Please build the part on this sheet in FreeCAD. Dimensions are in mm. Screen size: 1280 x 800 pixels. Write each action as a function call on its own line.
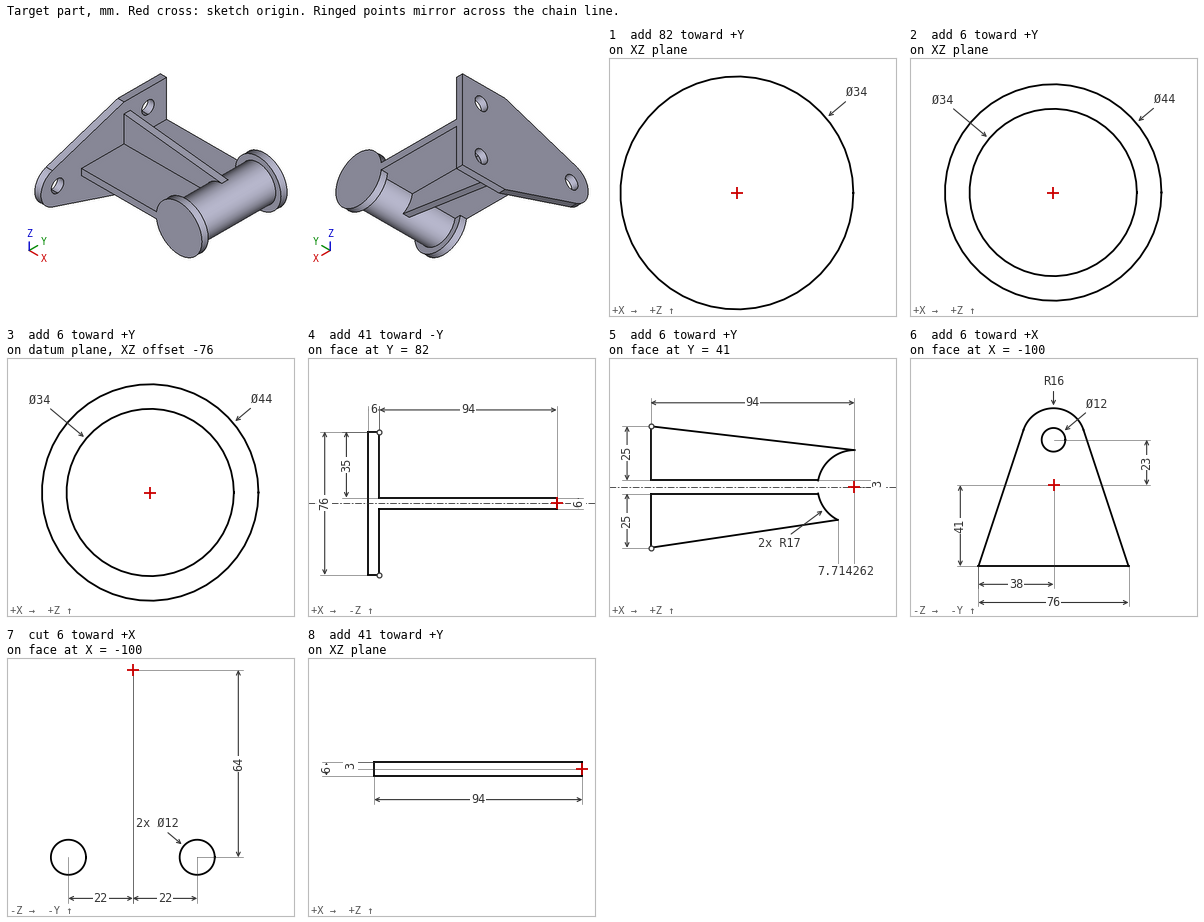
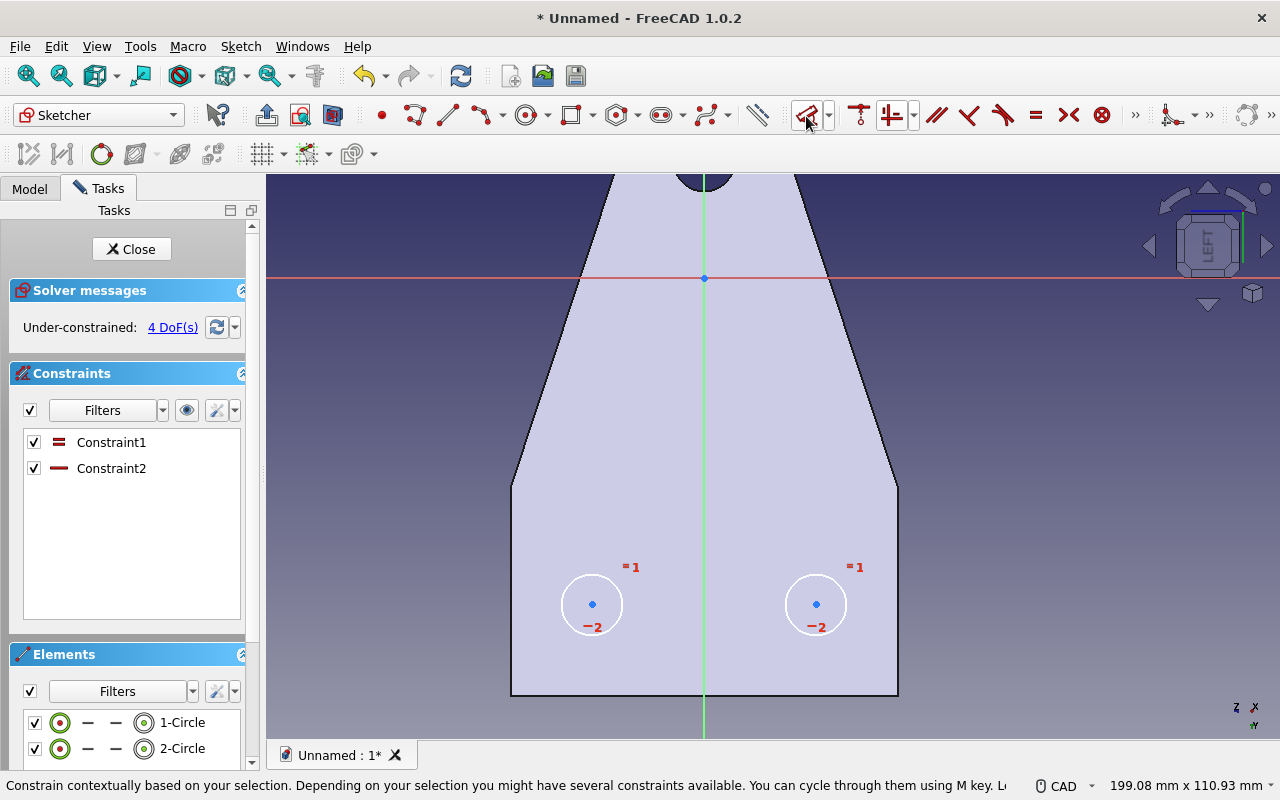
click(837, 583)
click(859, 560)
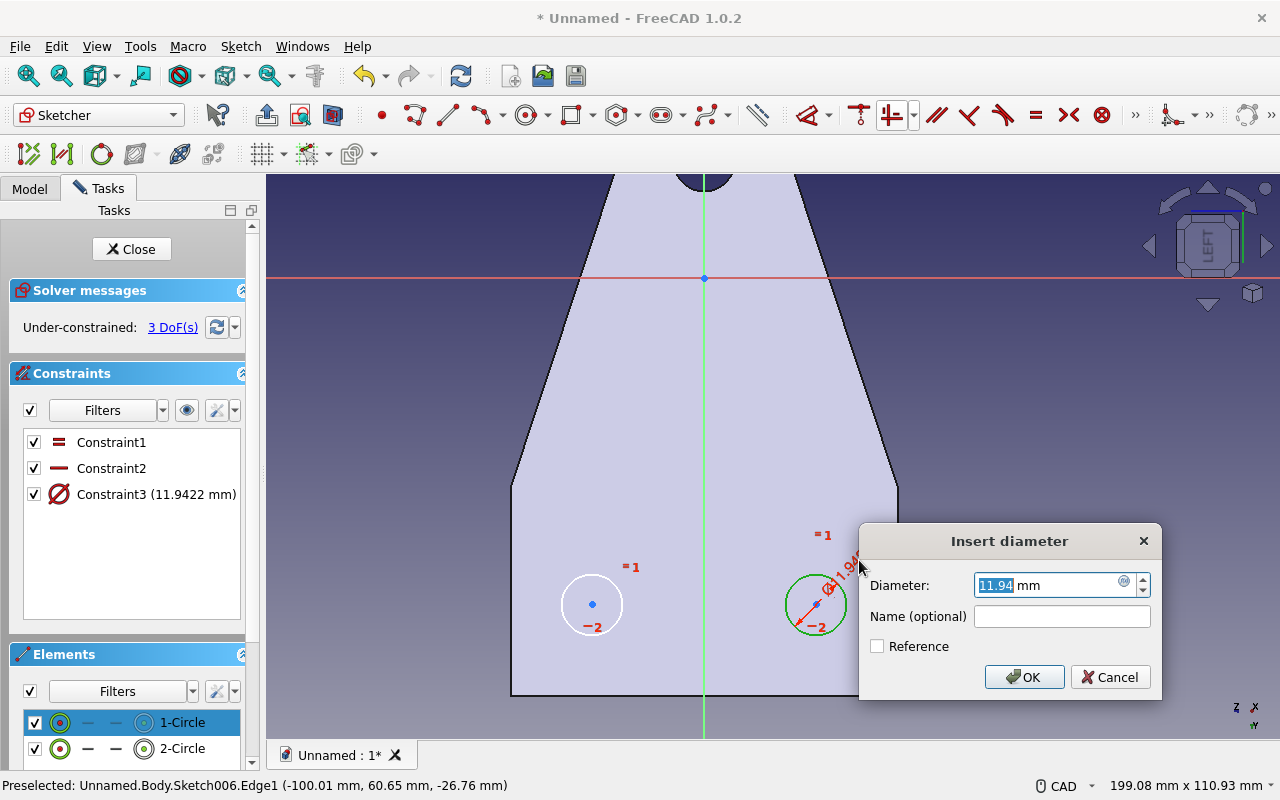
text(12)
key(Return)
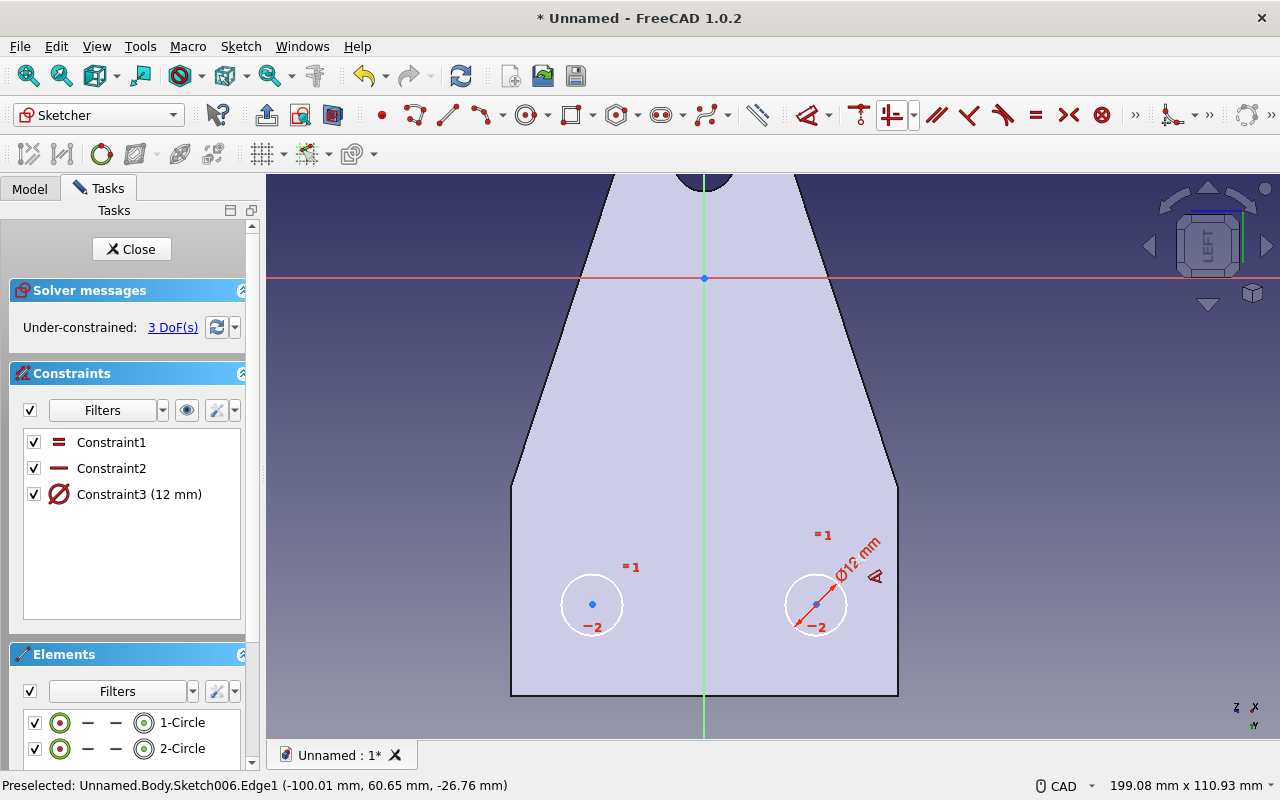
click(816, 605)
click(760, 244)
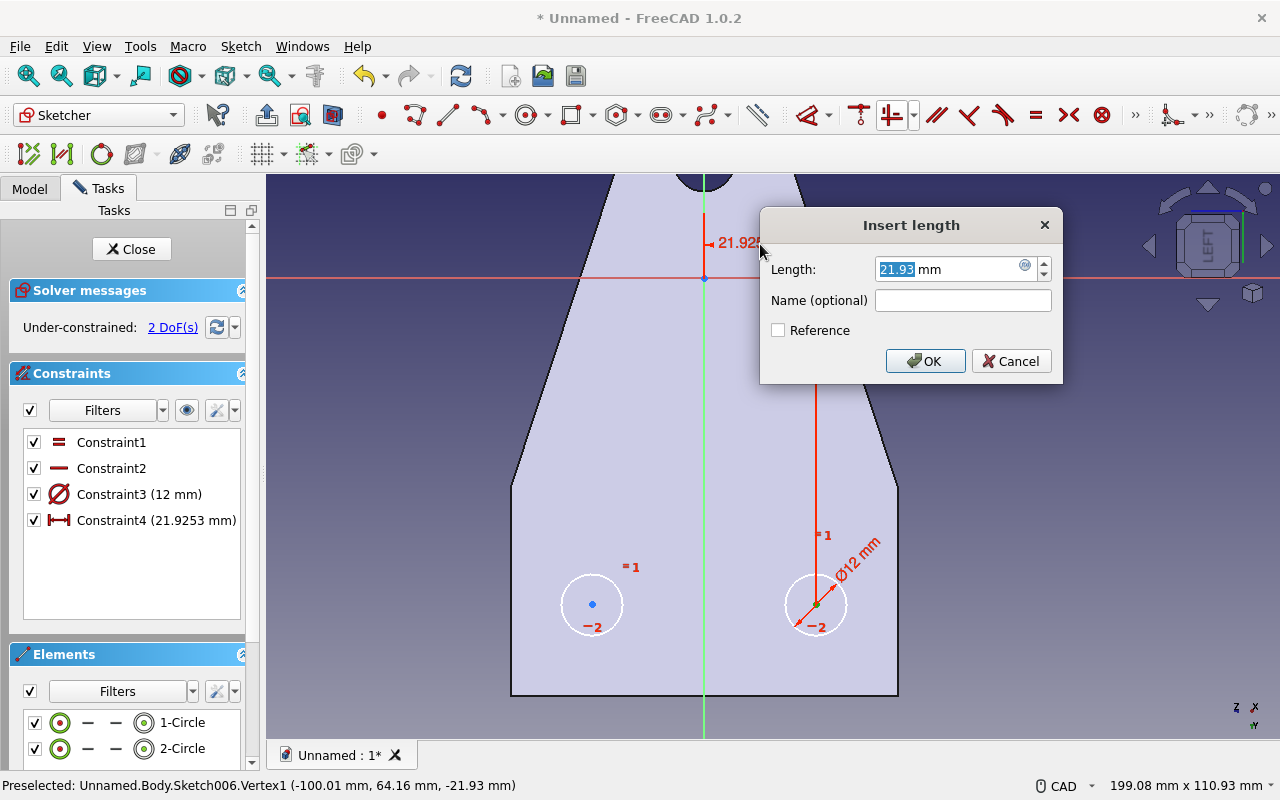
text(22)
key(Return)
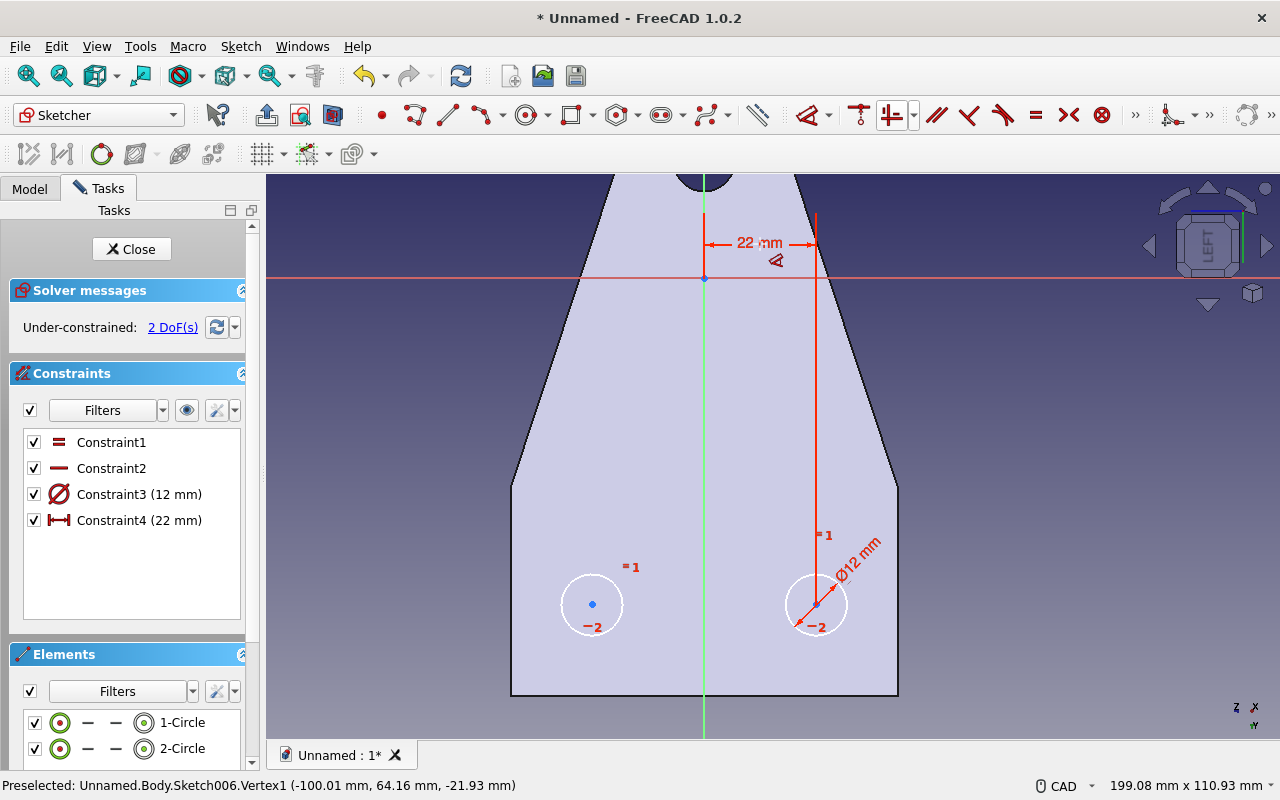
click(816, 605)
click(850, 442)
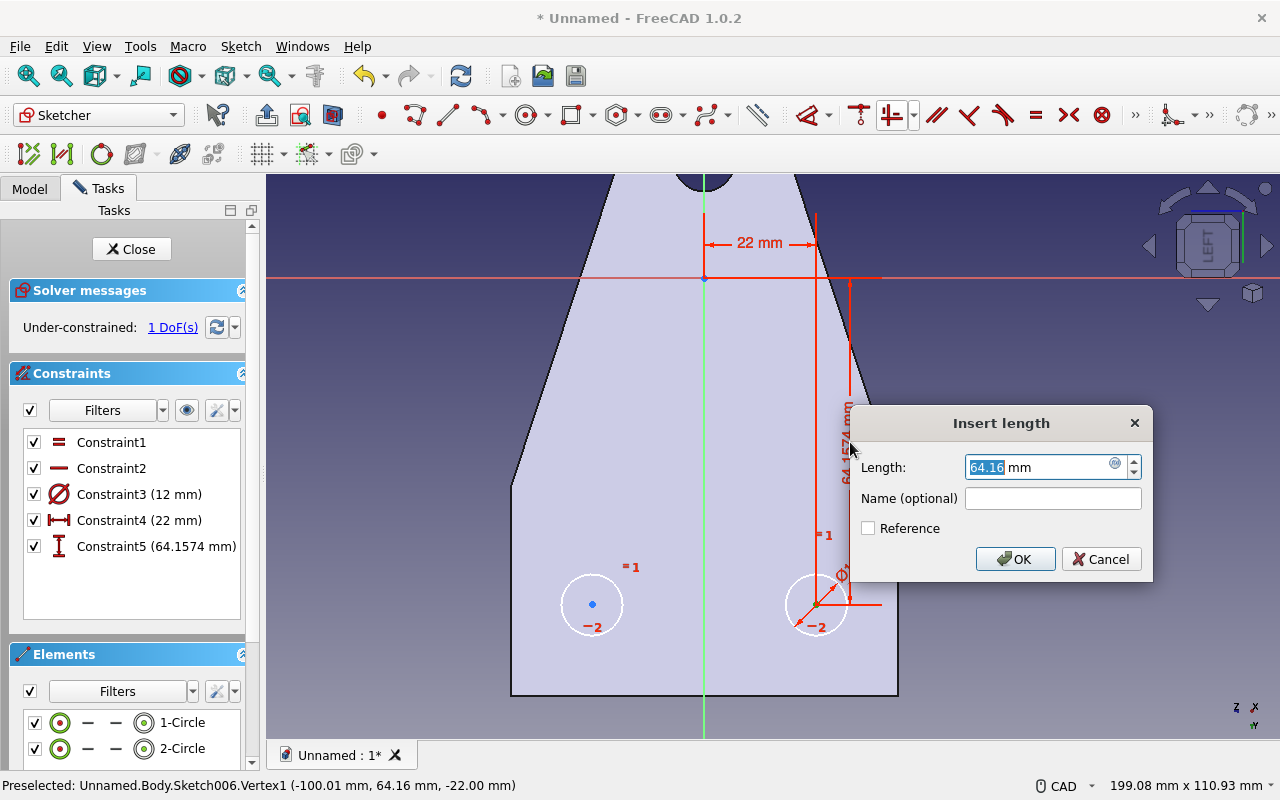
text(64)
key(Return)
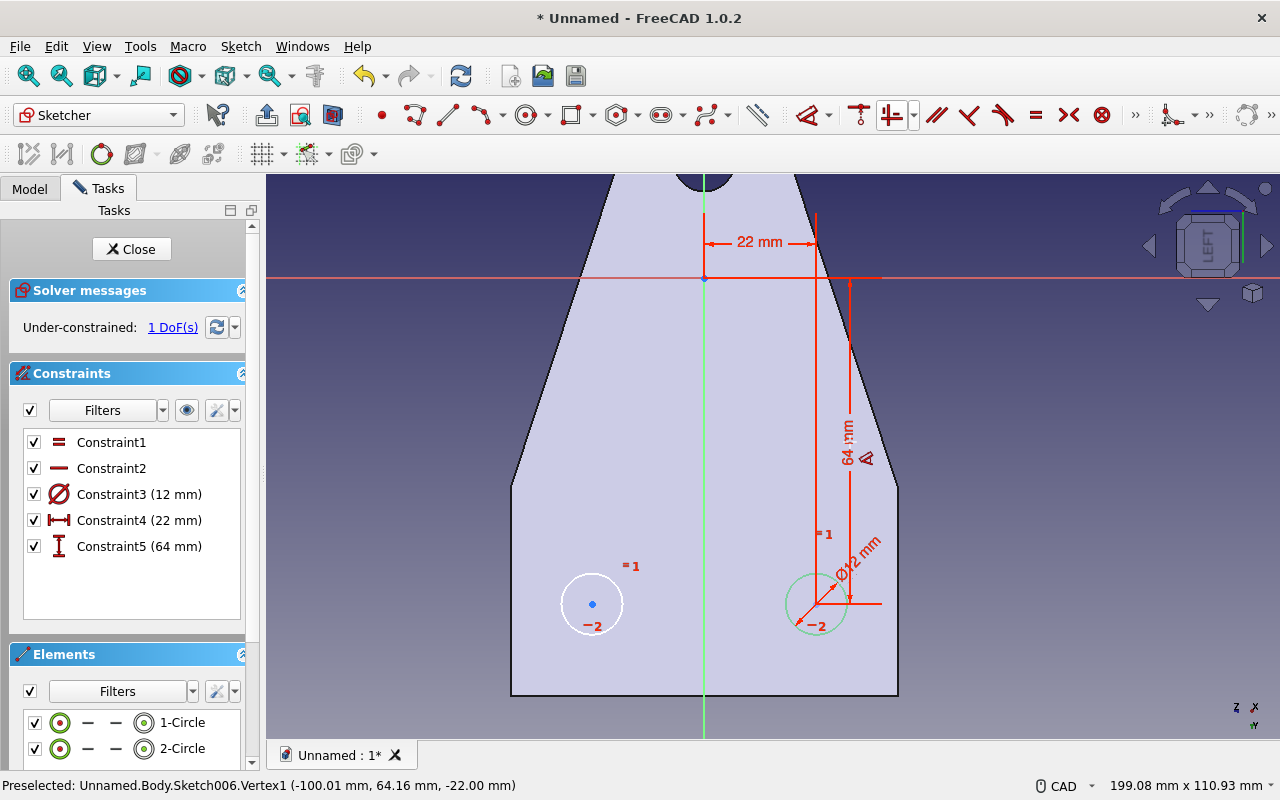
click(592, 604)
click(648, 244)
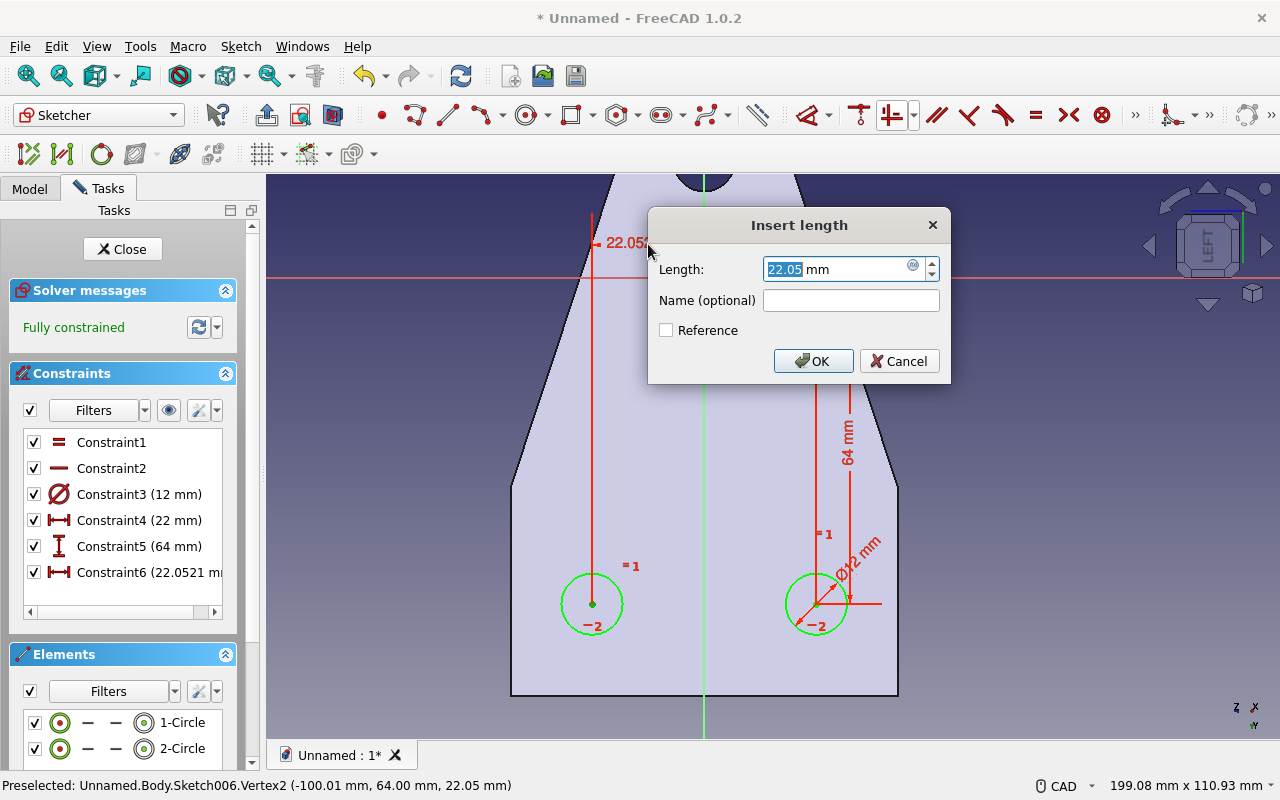
text(22)
key(Return)
key(Escape)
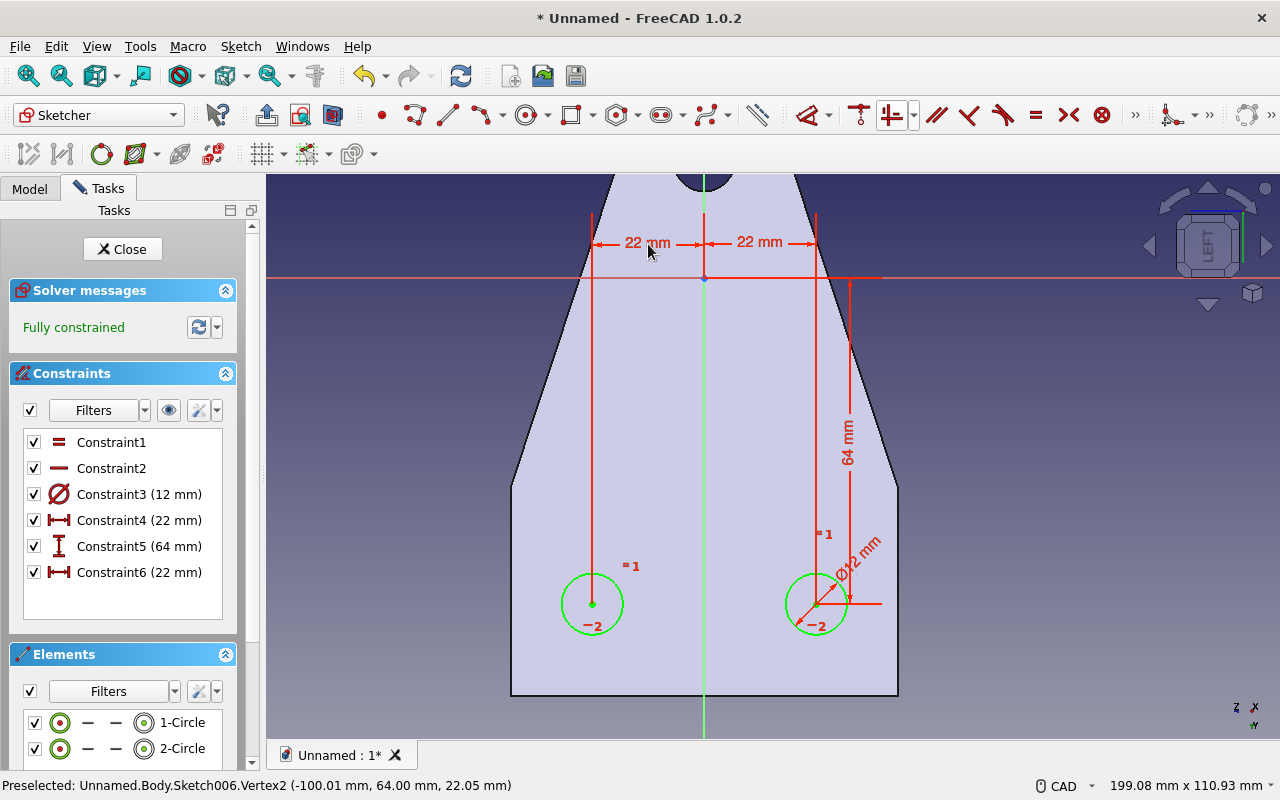
click(123, 249)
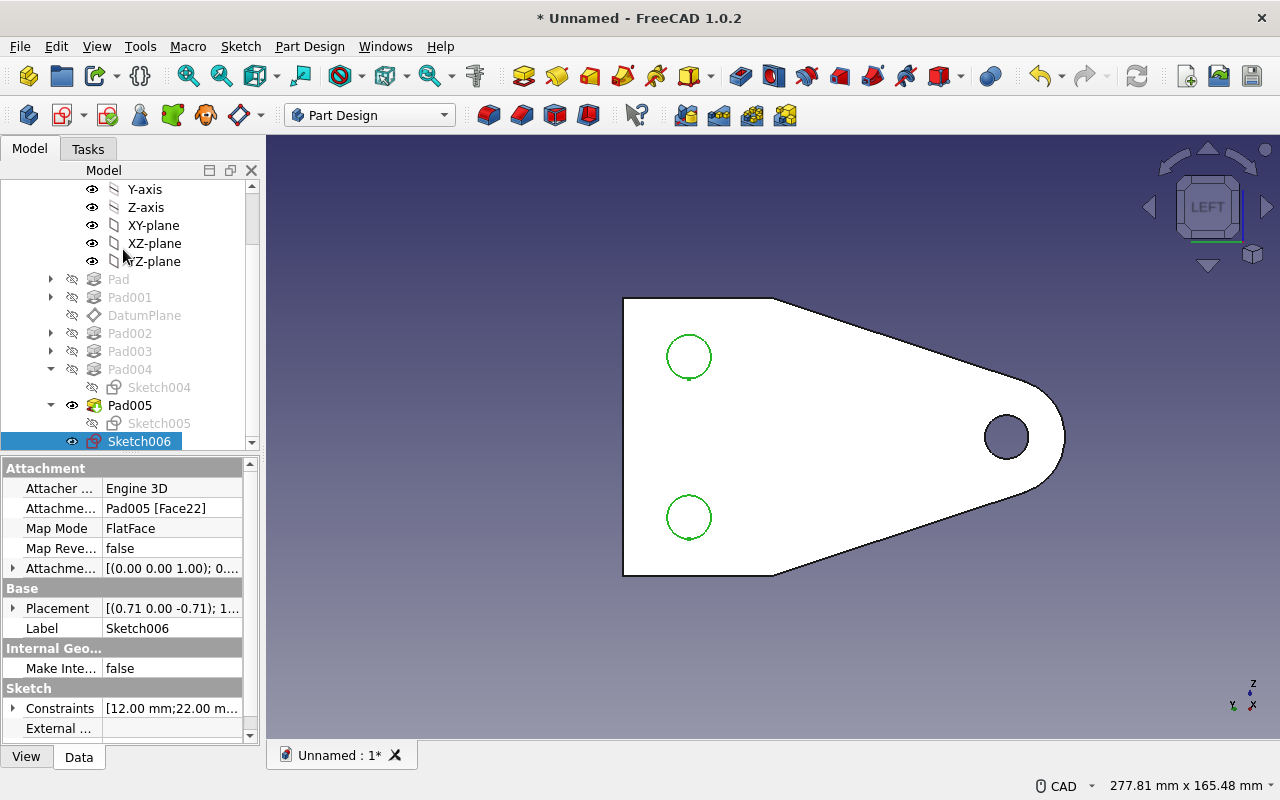
click(741, 76)